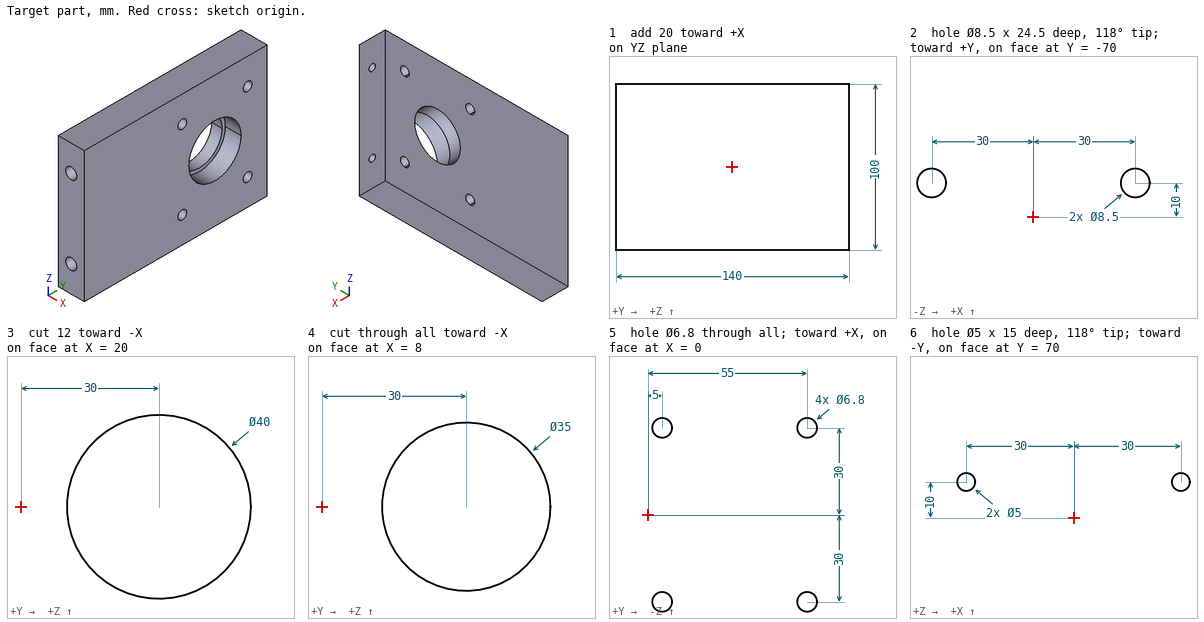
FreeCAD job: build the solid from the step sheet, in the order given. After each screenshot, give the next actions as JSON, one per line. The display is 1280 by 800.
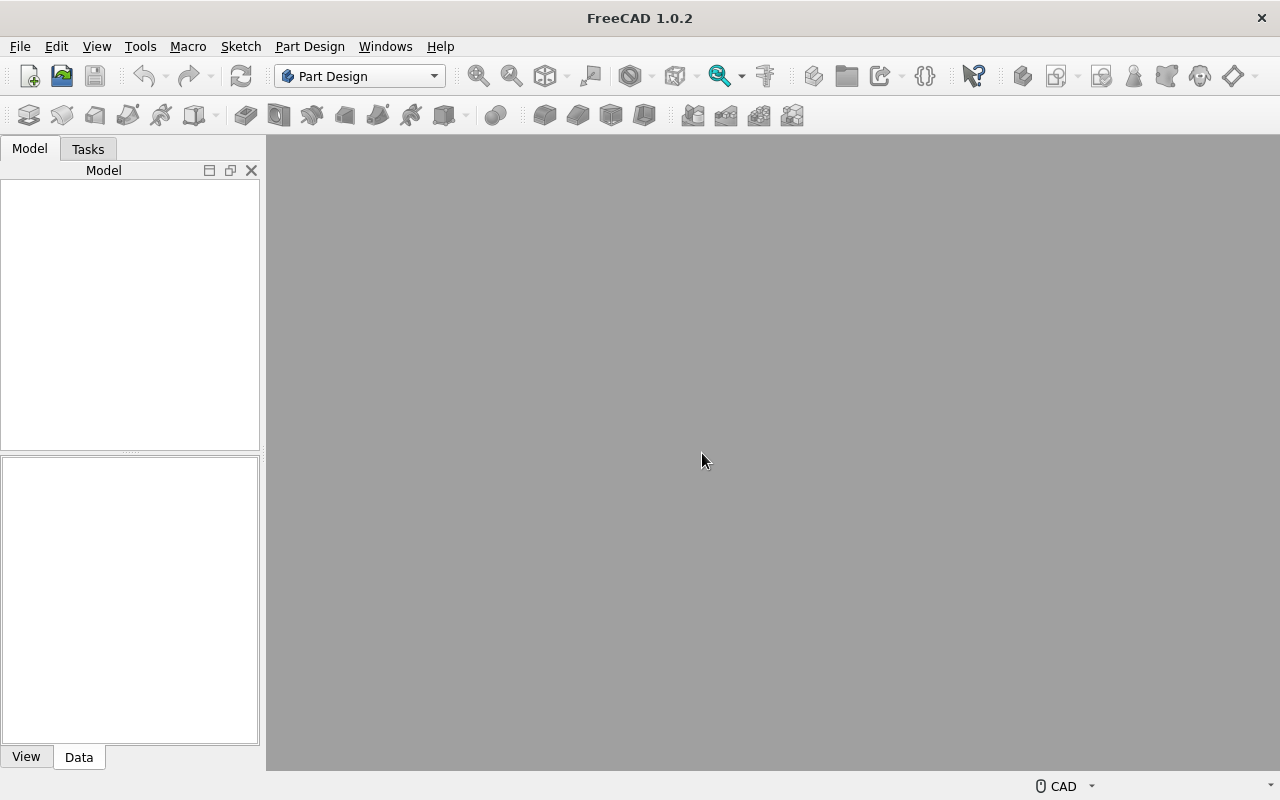
{"action": "key", "text": "ctrl+n"}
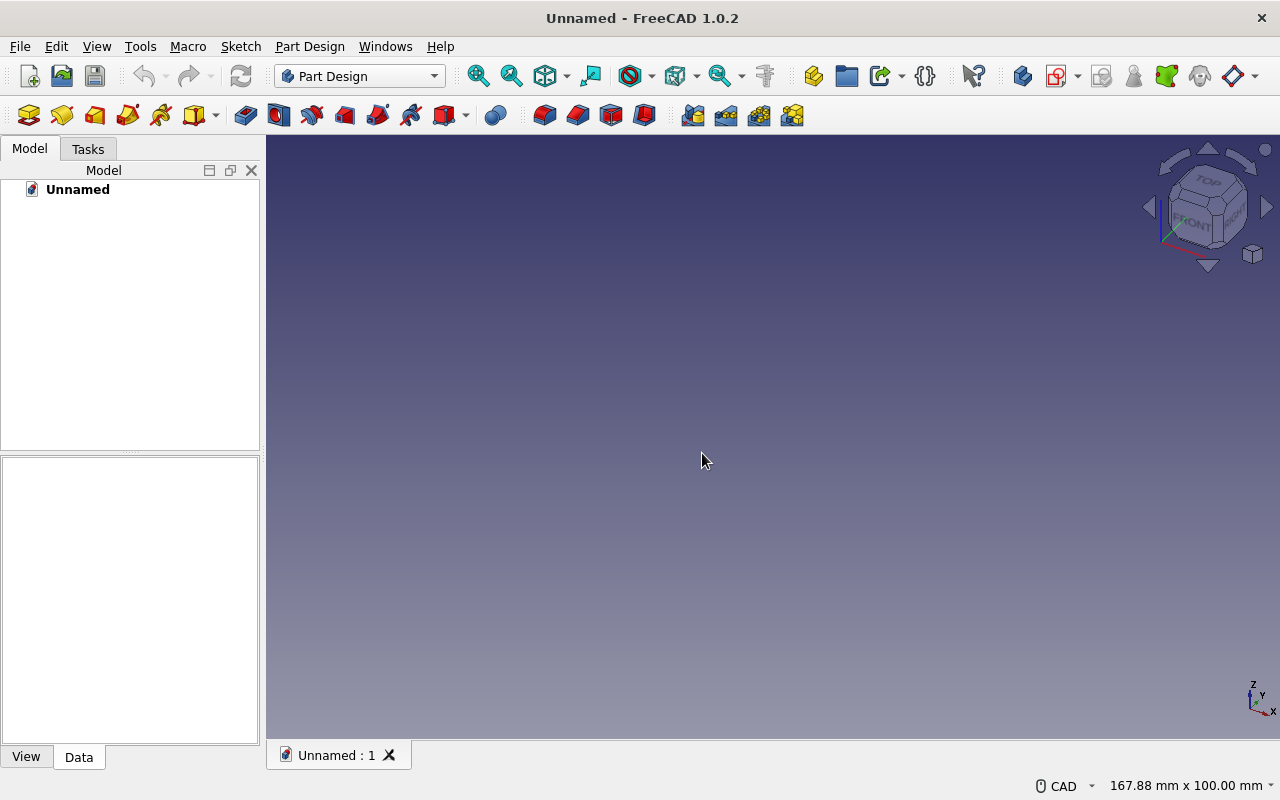
{"action": "left_click", "coordinate": [1056, 76]}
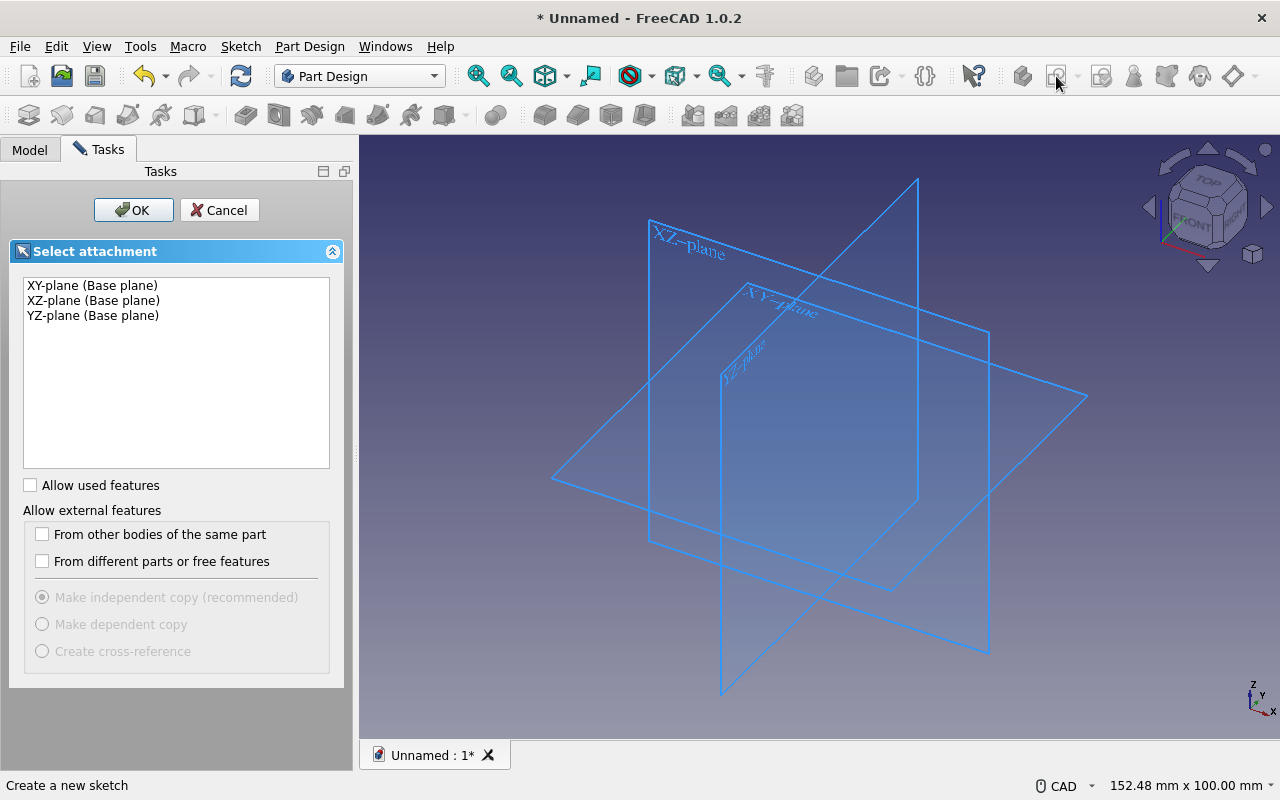
{"action": "left_click", "coordinate": [84, 316]}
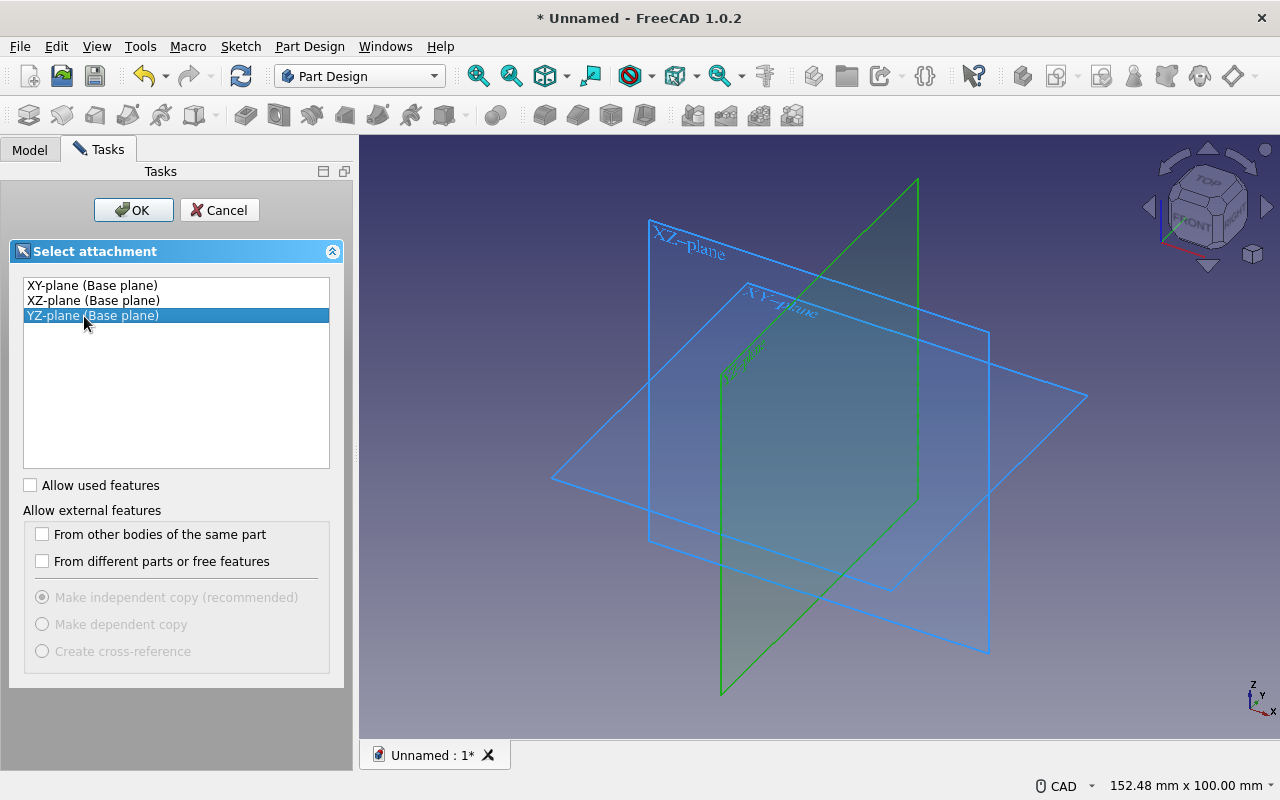
{"action": "left_click", "coordinate": [134, 210]}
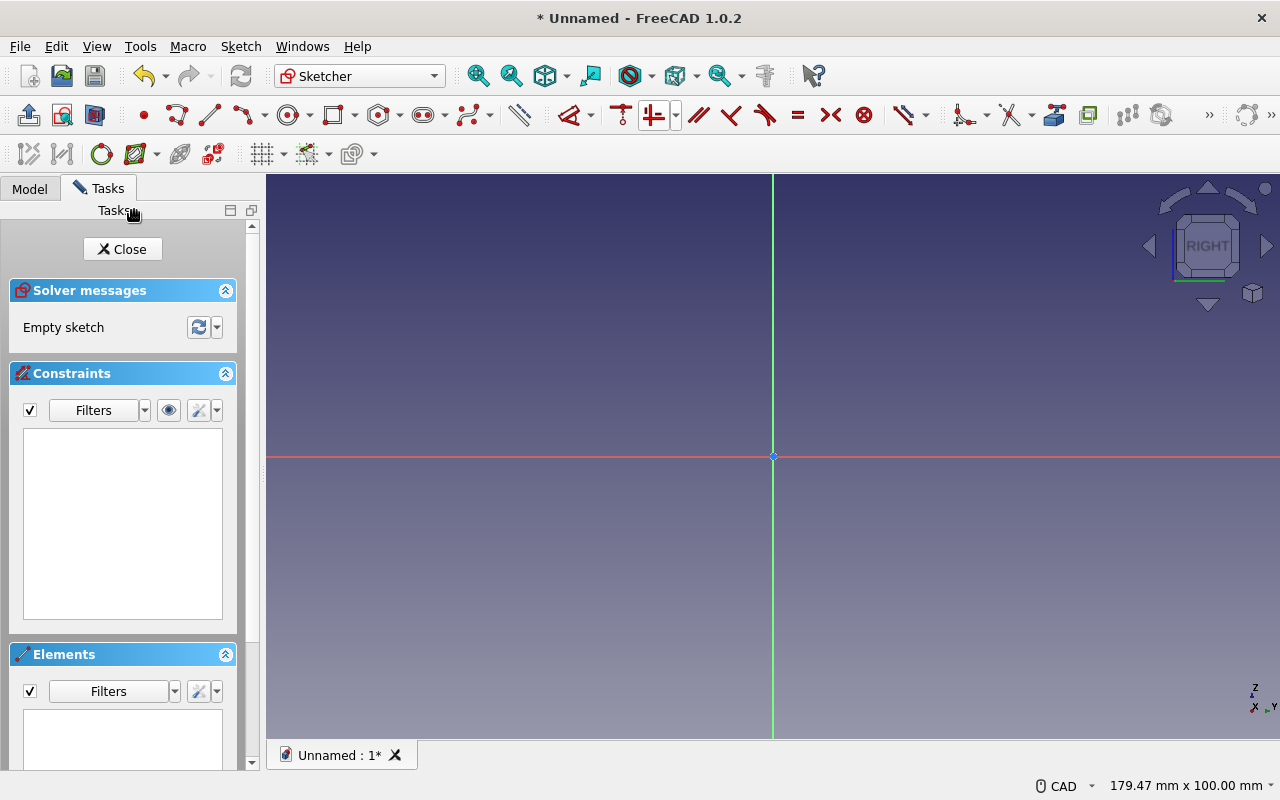
{"action": "scroll", "coordinate": [565, 457], "scroll_direction": "down", "scroll_amount": 2}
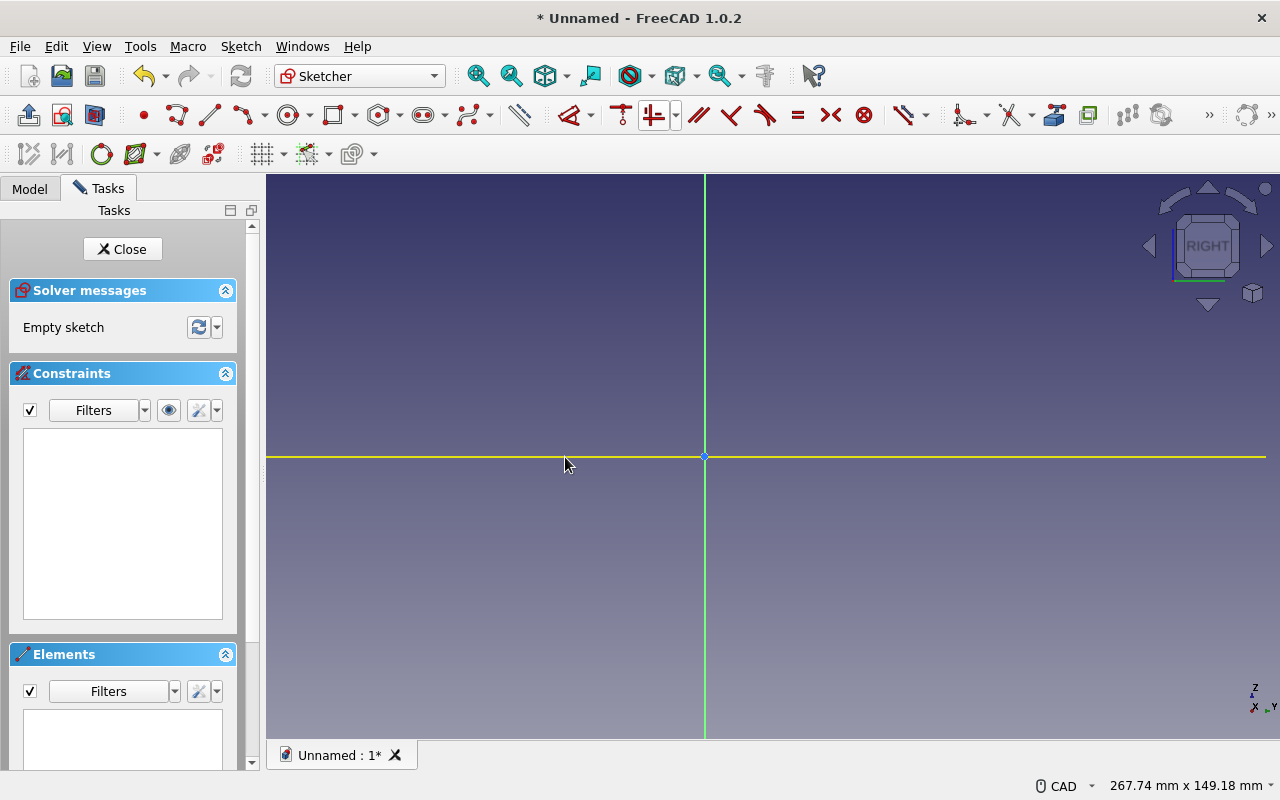
{"action": "key", "text": "g v"}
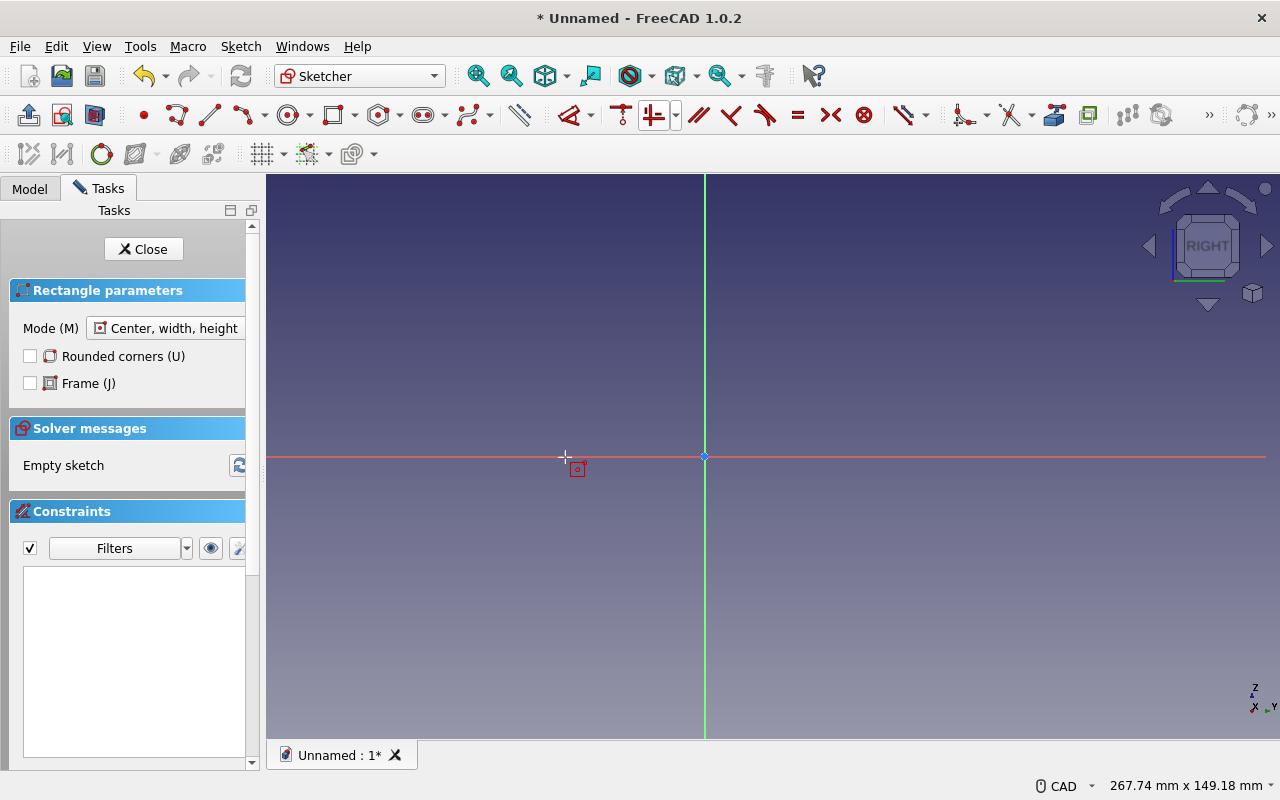
{"action": "left_click", "coordinate": [705, 457]}
{"action": "mouse_move", "coordinate": [970, 267]}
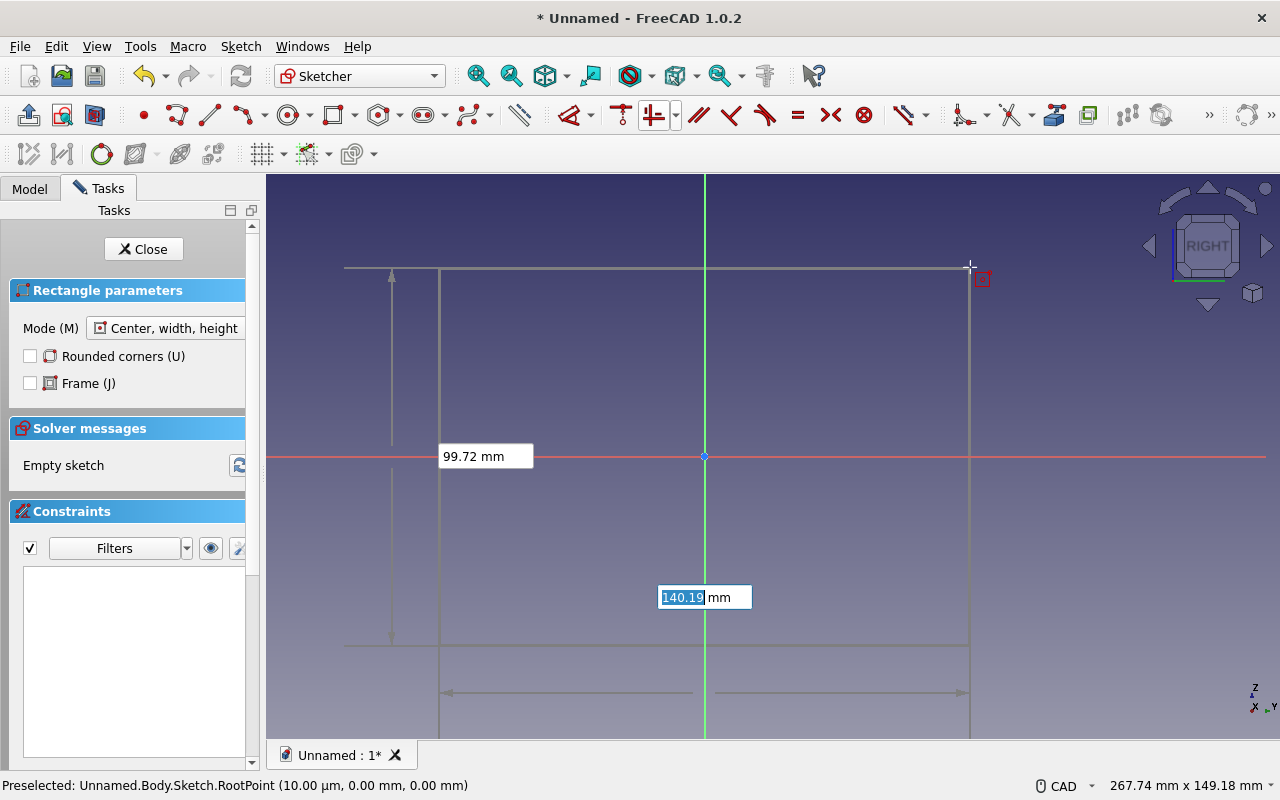
{"action": "type", "text": "140"}
{"action": "key", "text": "Tab"}
{"action": "type", "text": "100"}
{"action": "key", "text": "Return"}
{"action": "key", "text": "Escape"}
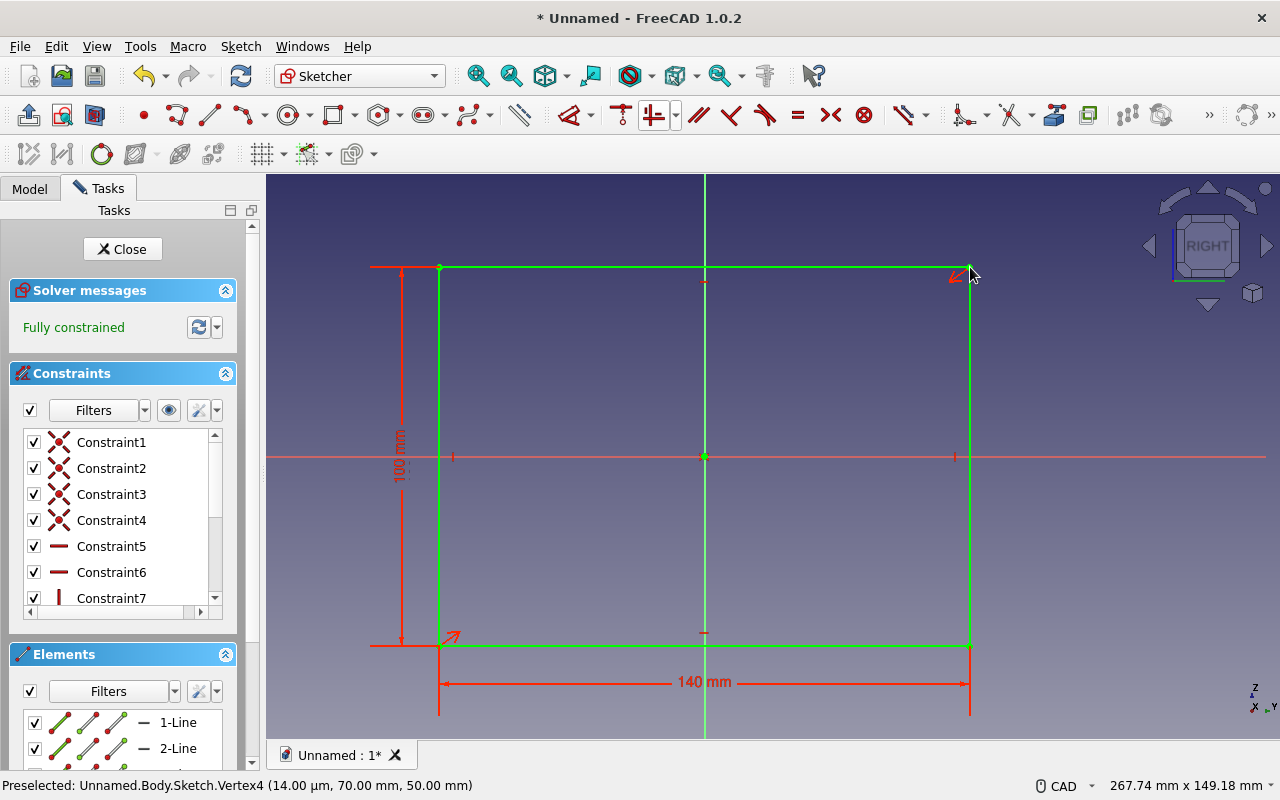
{"action": "left_click", "coordinate": [123, 249]}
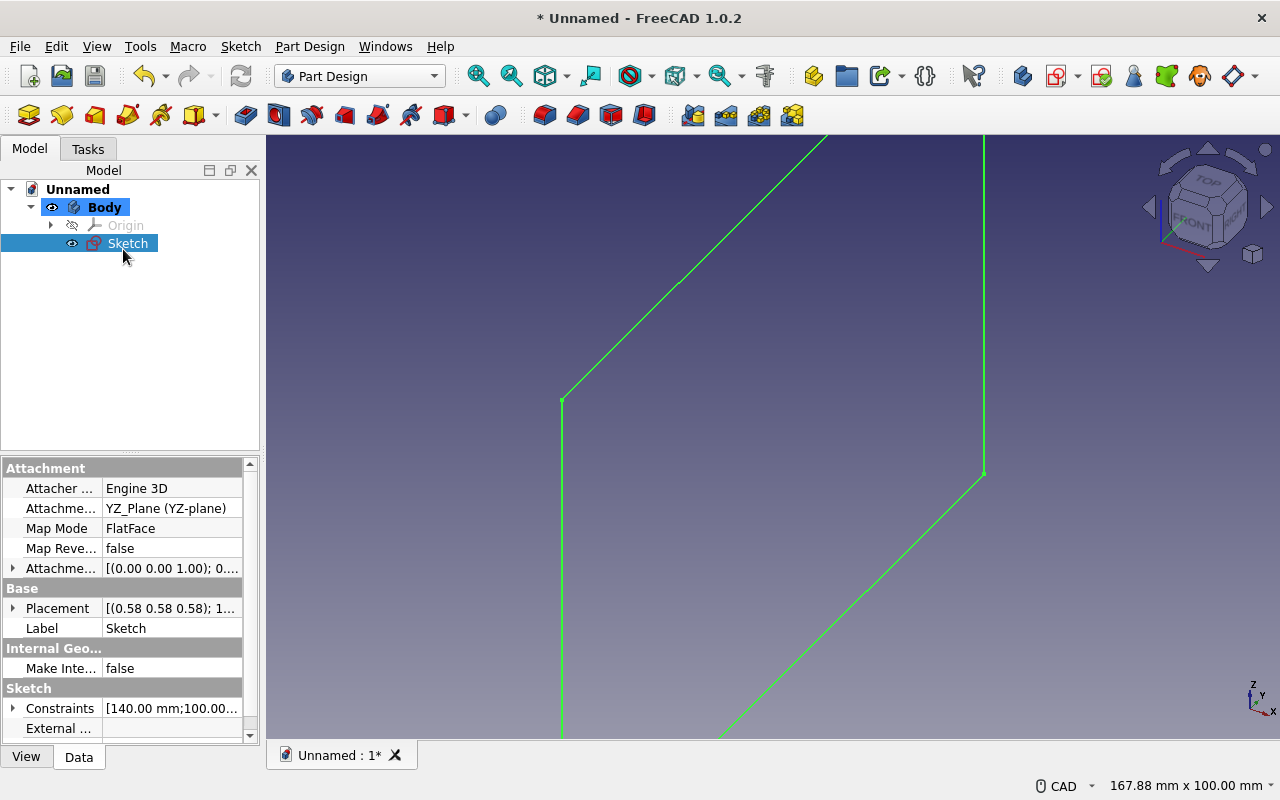
{"action": "left_click", "coordinate": [29, 116]}